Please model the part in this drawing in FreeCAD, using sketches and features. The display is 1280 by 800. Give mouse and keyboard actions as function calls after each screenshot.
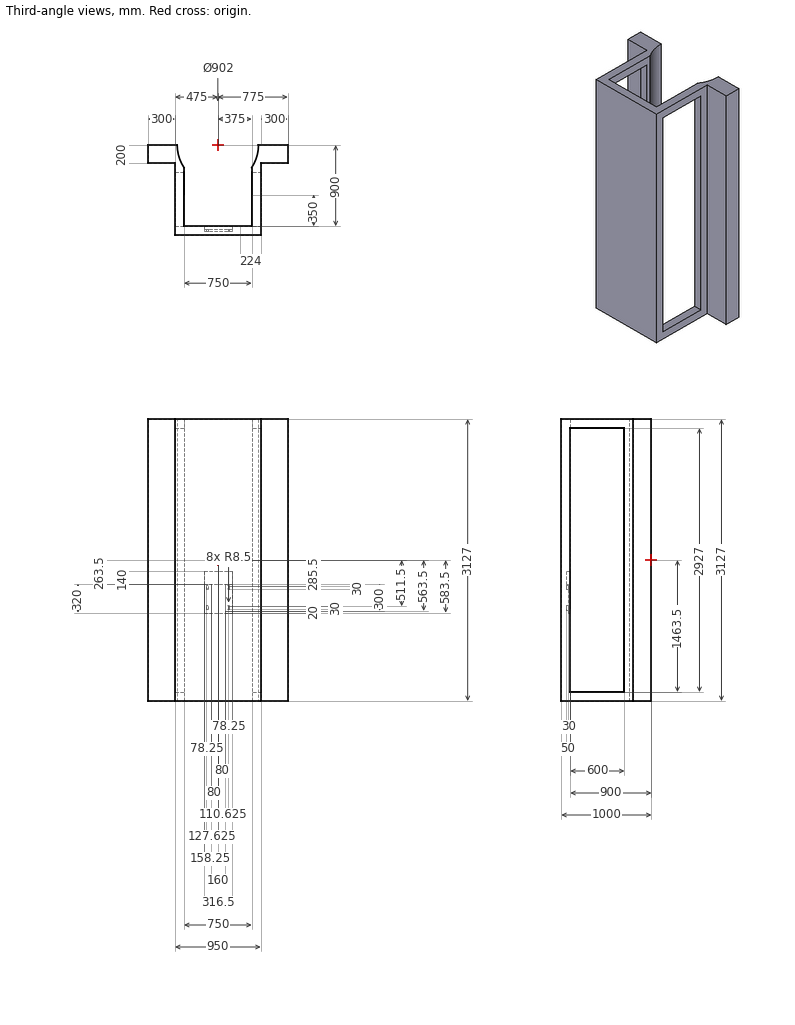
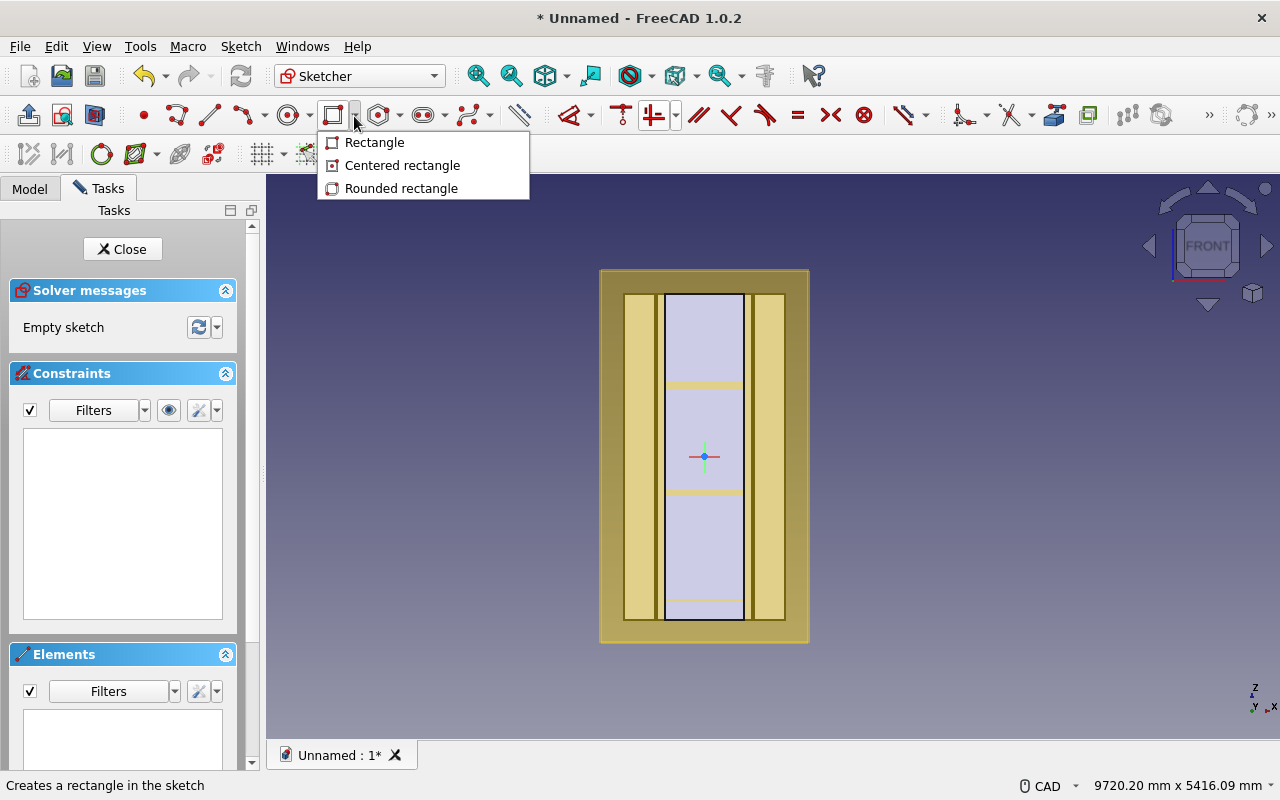
click(424, 166)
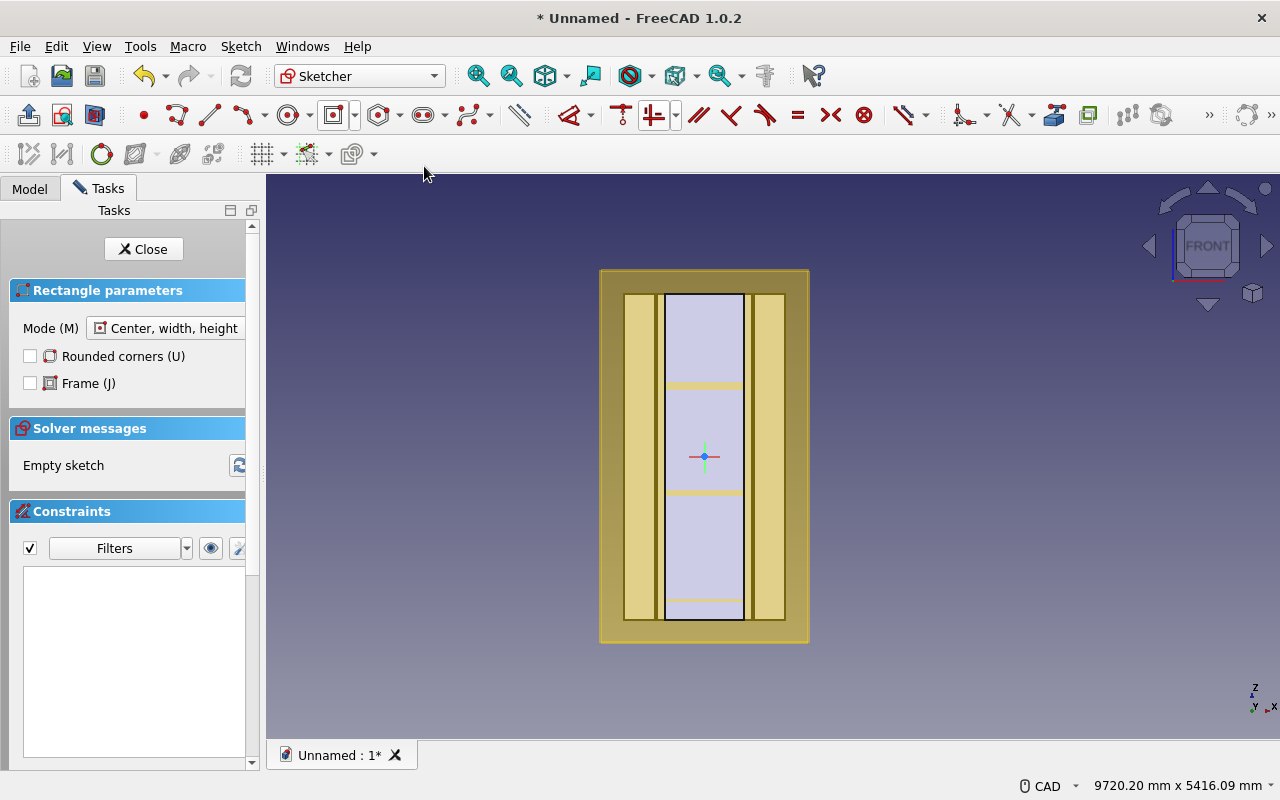
click(705, 457)
click(744, 294)
key(Escape)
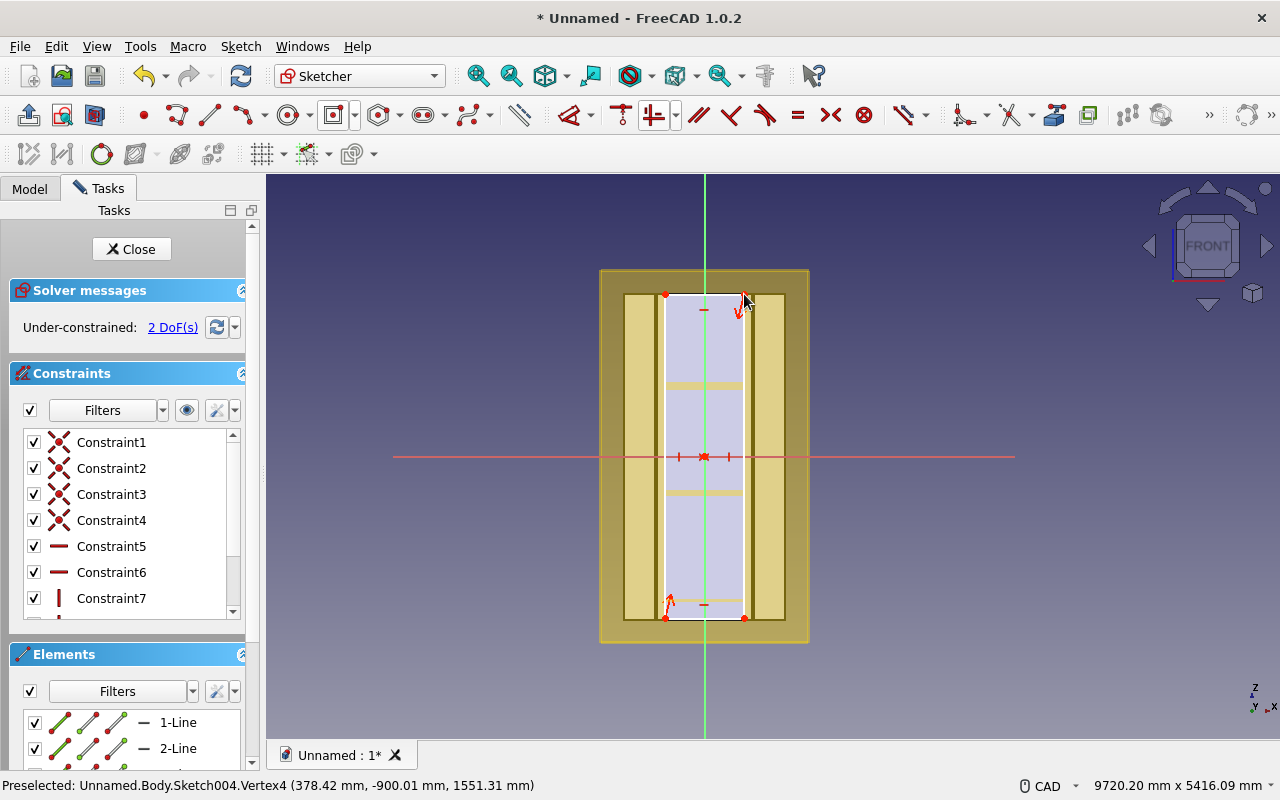
click(568, 116)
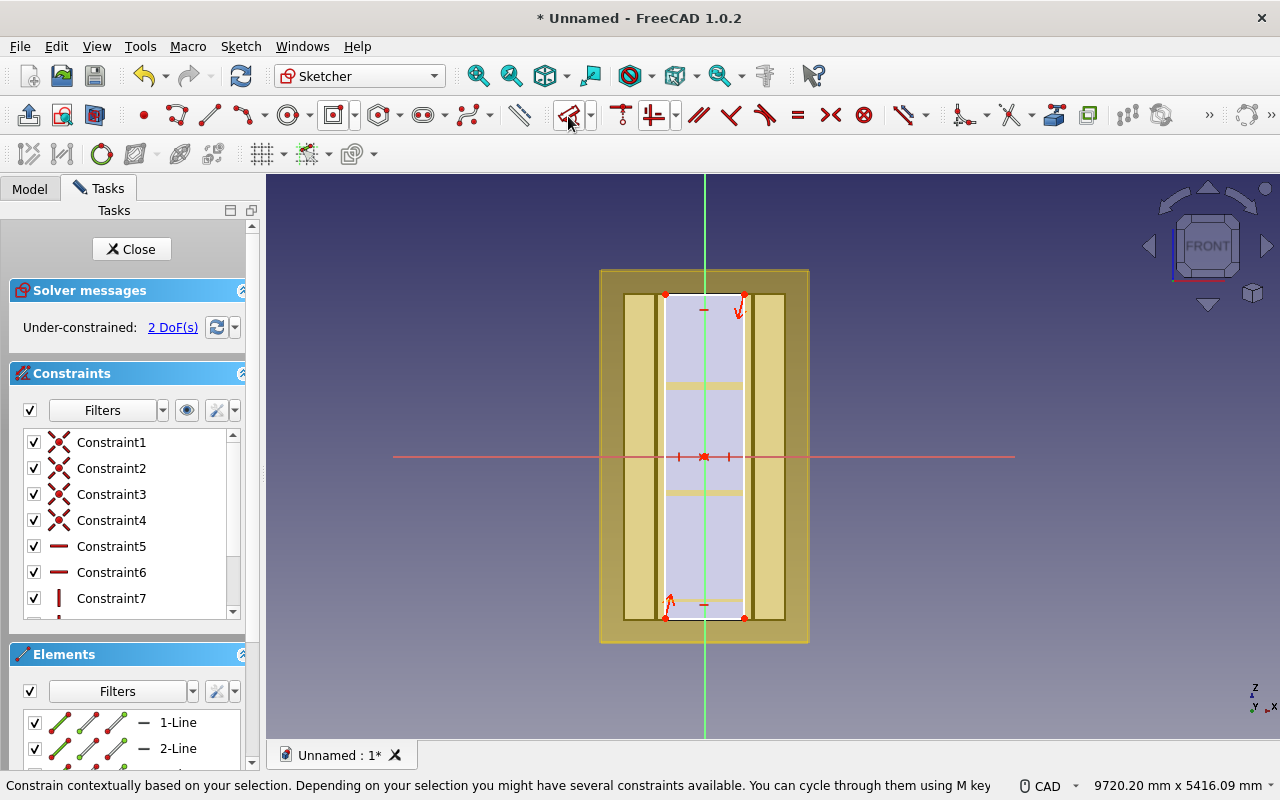
click(689, 619)
click(686, 653)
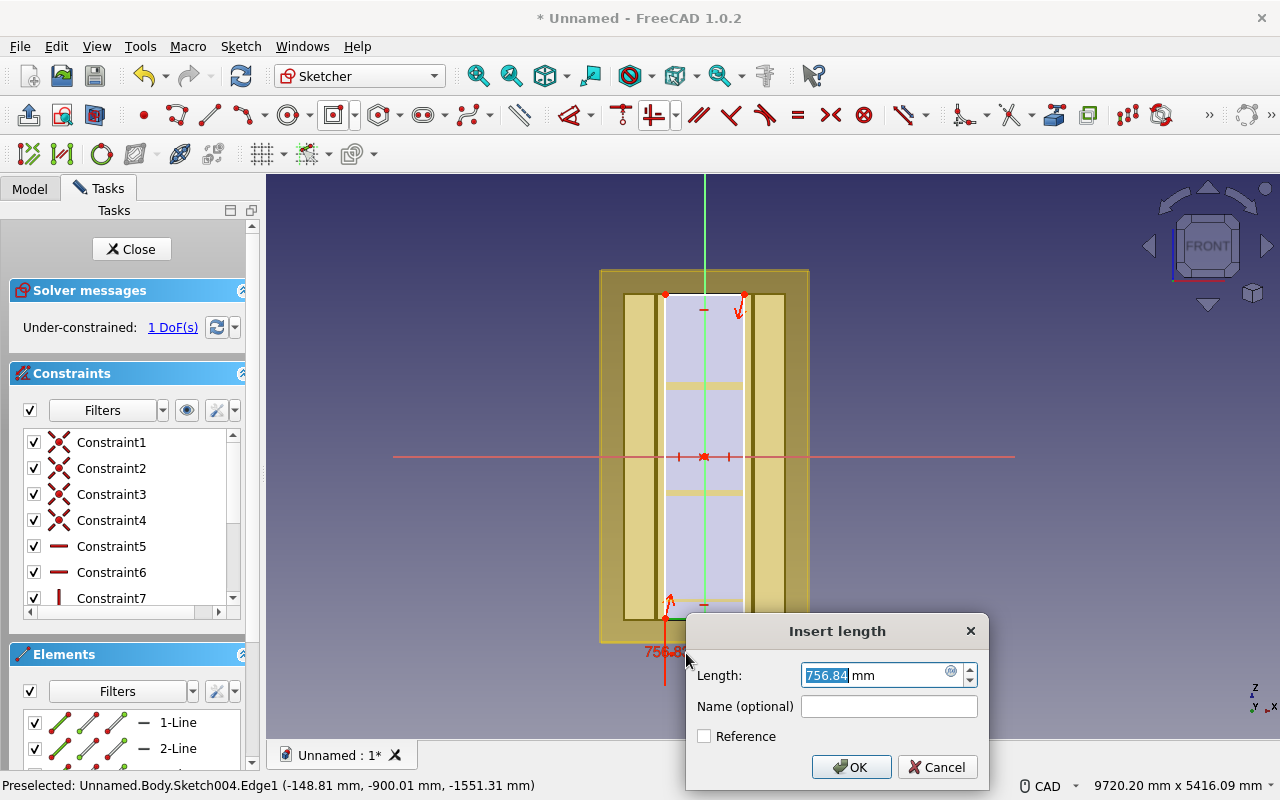
text(750)
key(Return)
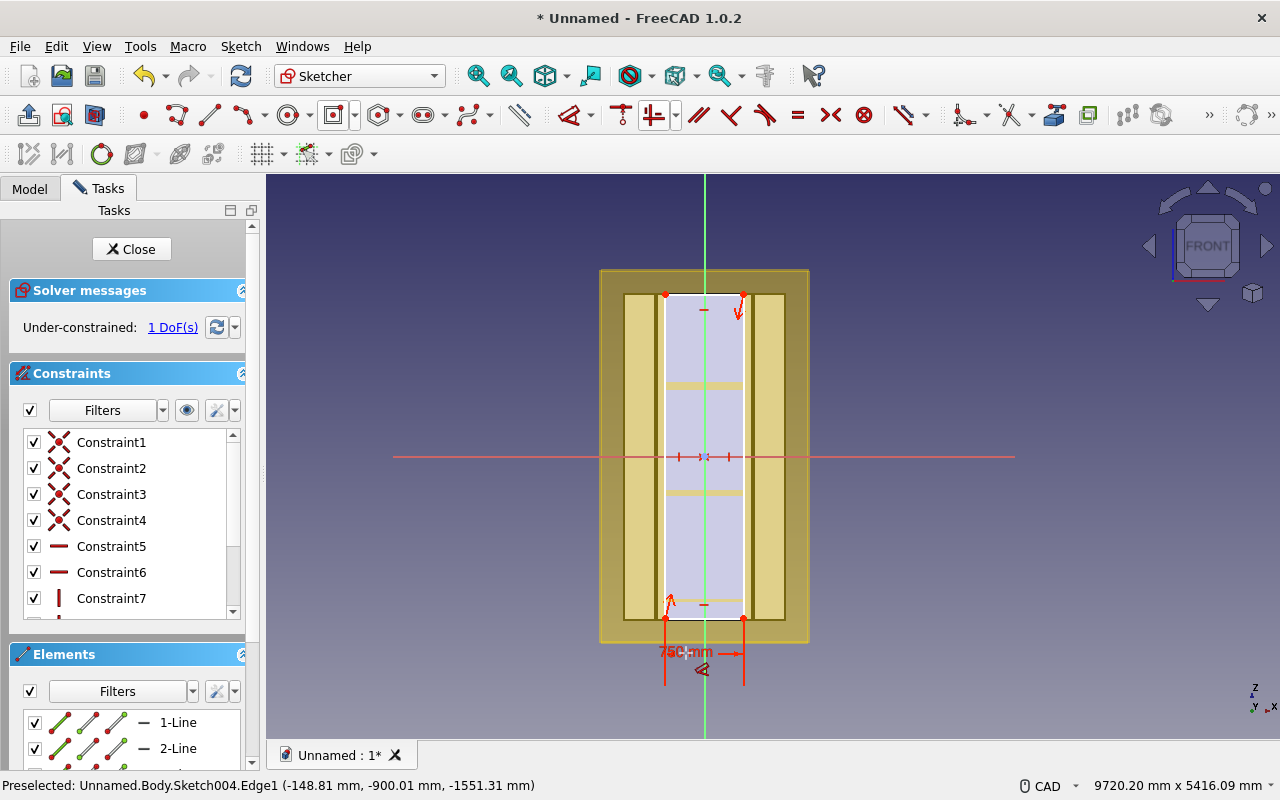
click(744, 522)
click(778, 382)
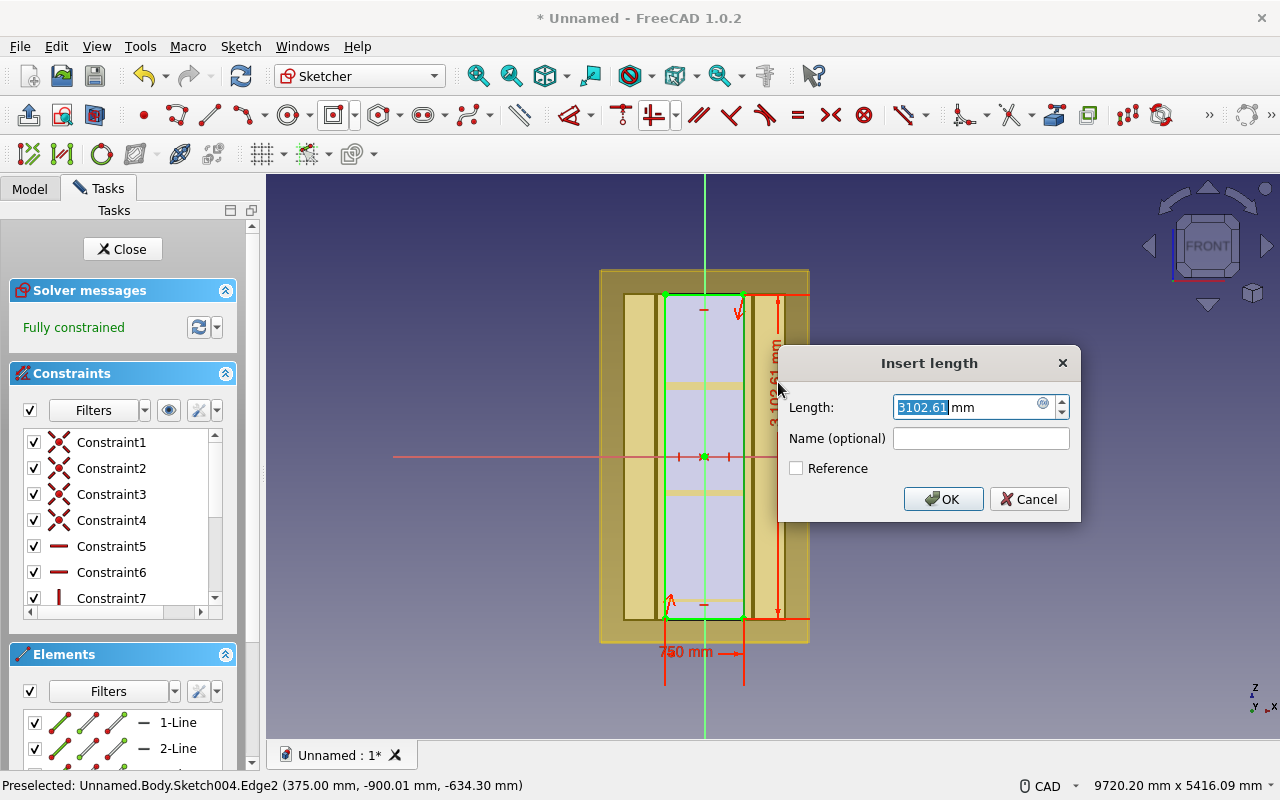
text(3127)
key(Return)
key(Escape)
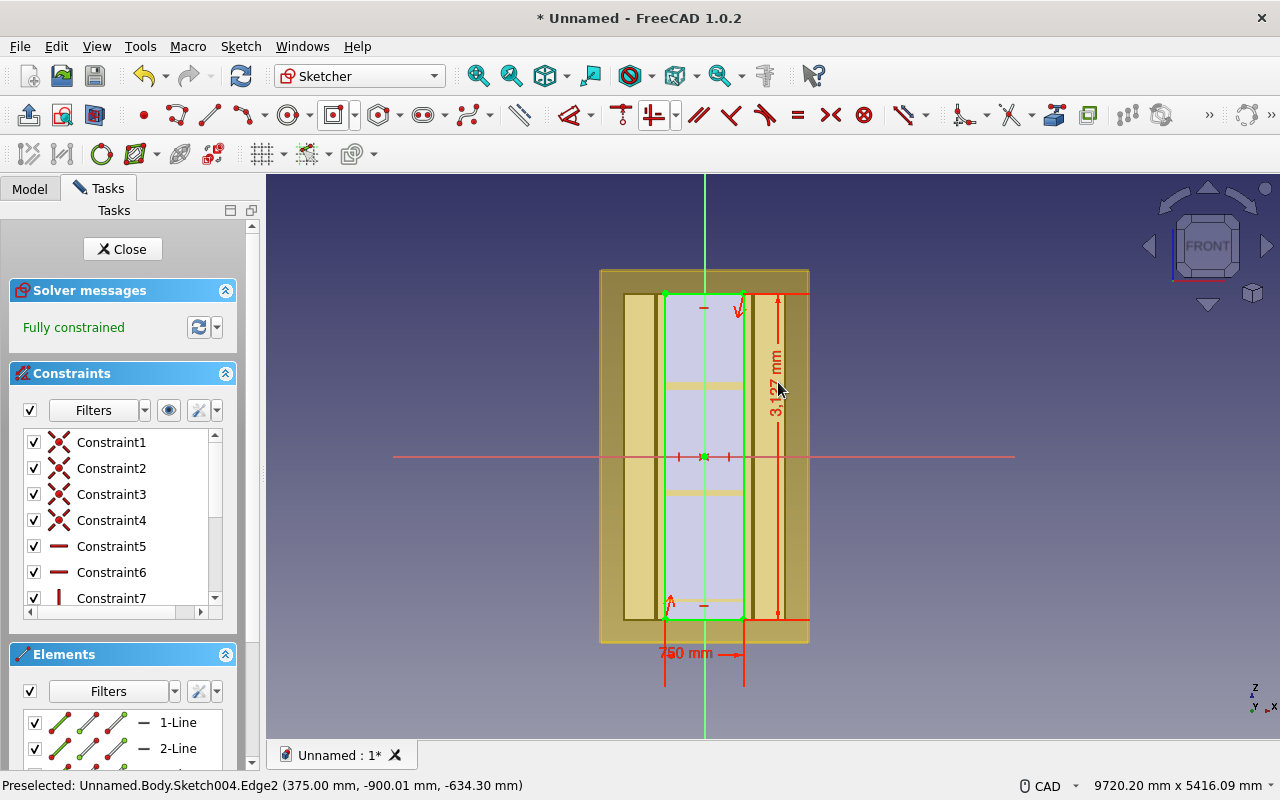
click(123, 249)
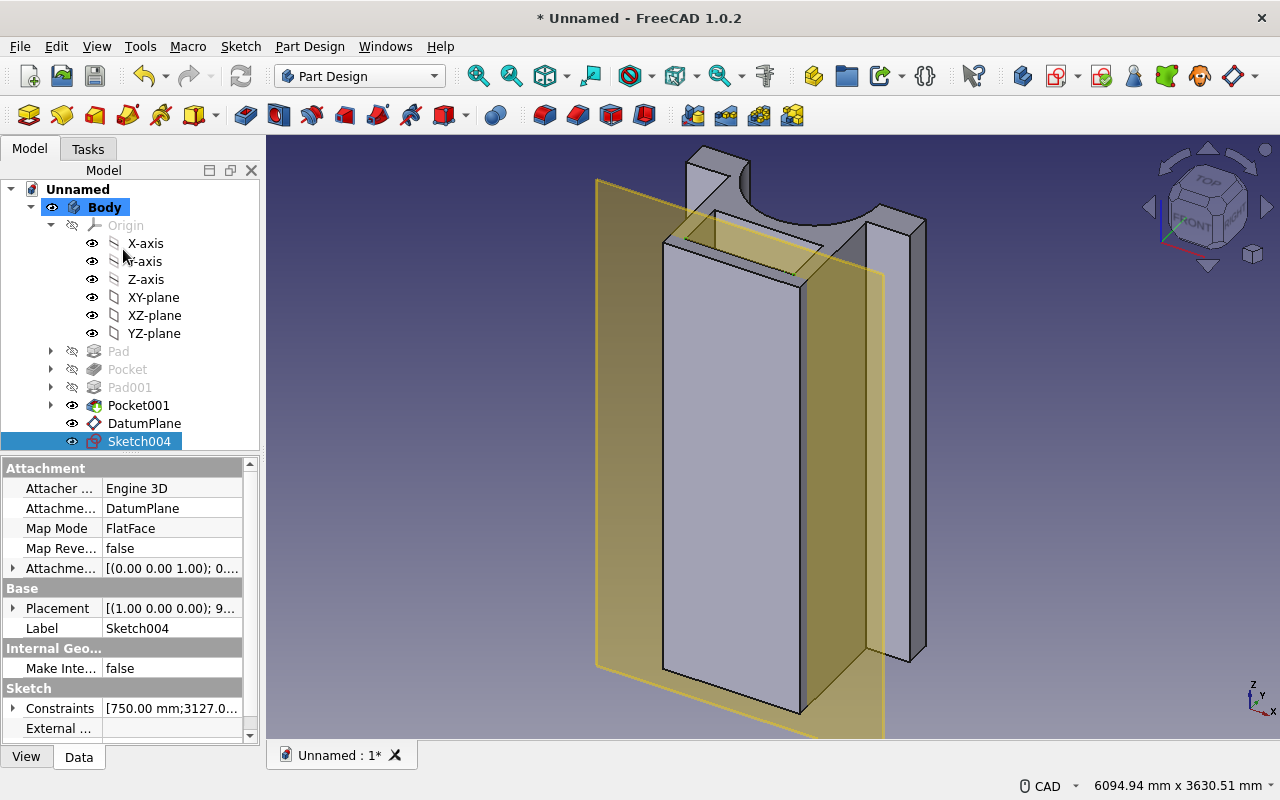
click(246, 116)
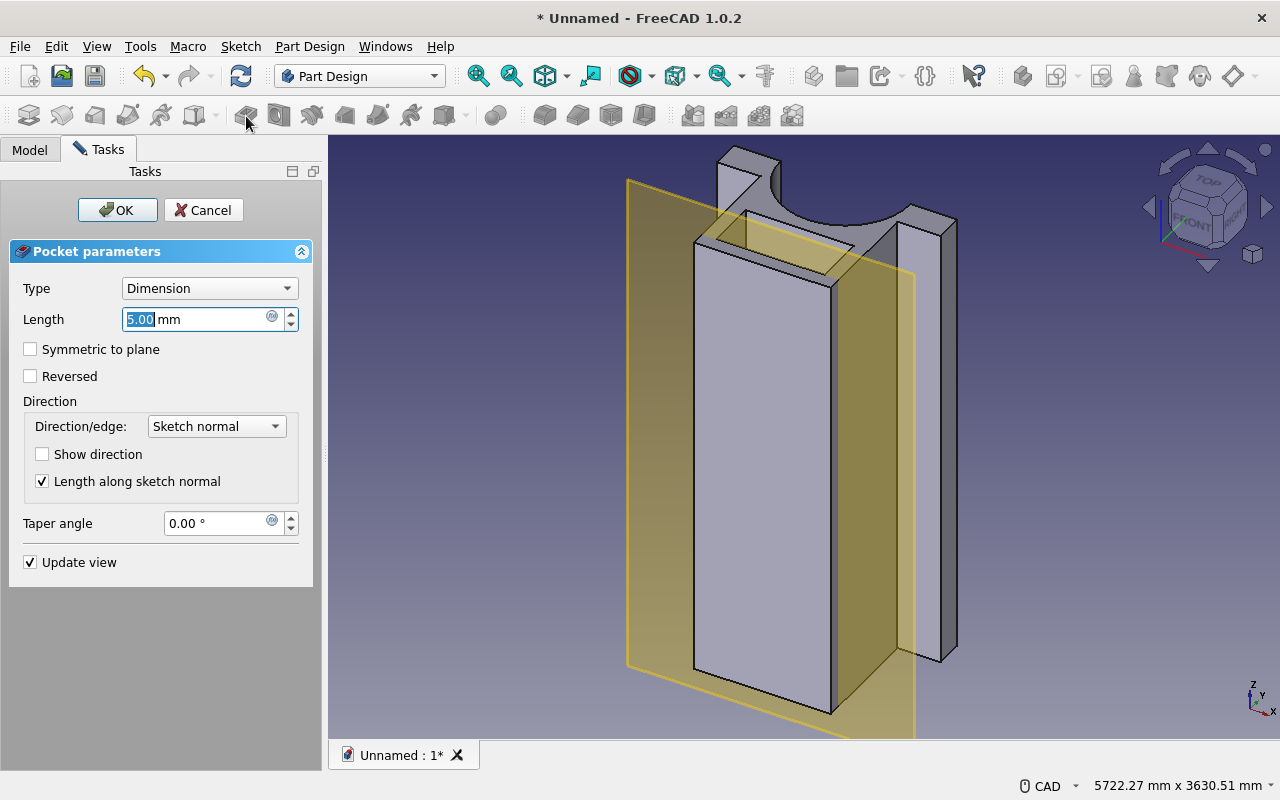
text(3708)
key(Tab)